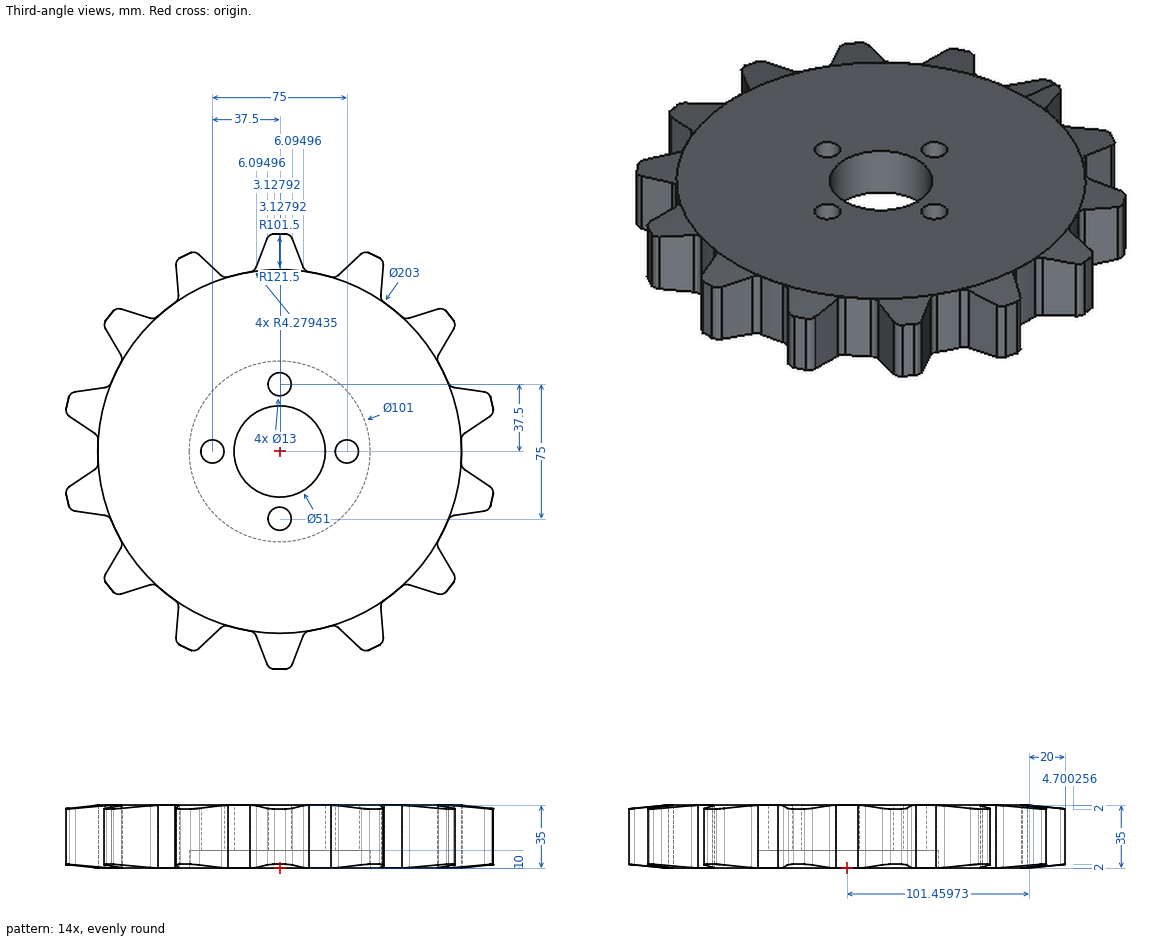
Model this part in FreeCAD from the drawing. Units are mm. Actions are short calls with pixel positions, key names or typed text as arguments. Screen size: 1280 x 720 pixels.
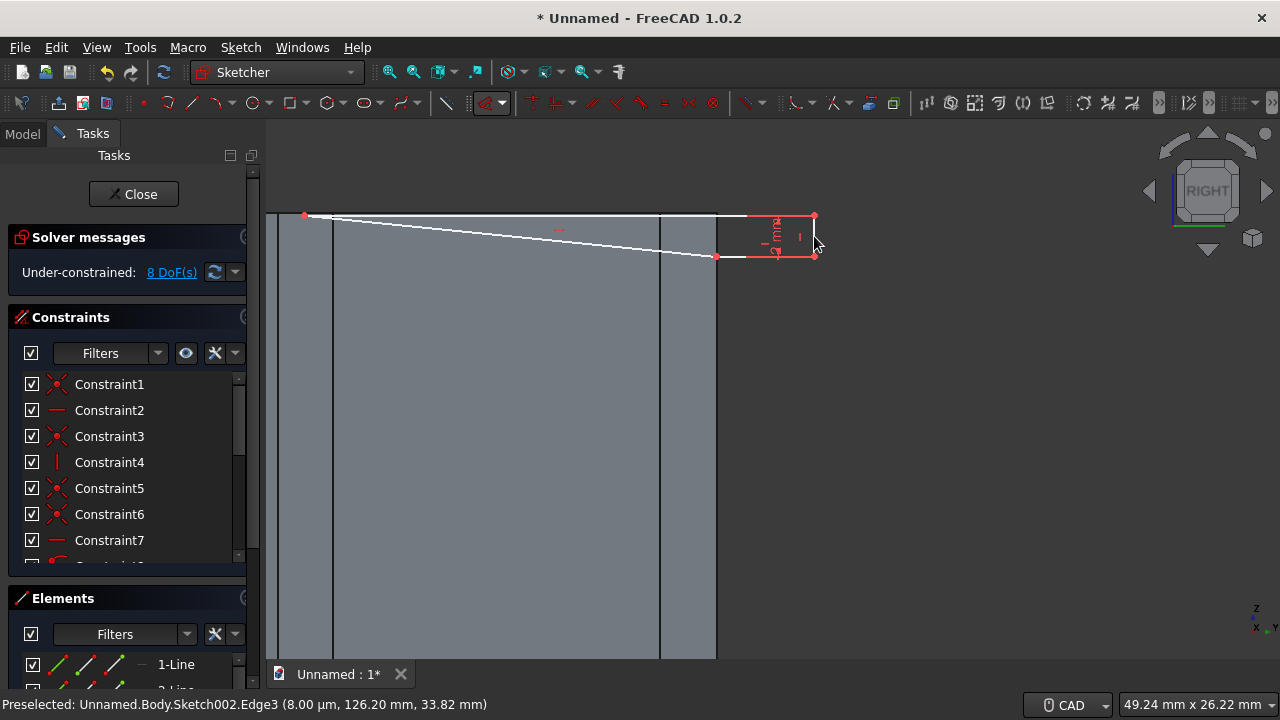
scroll(823, 239, down, 4)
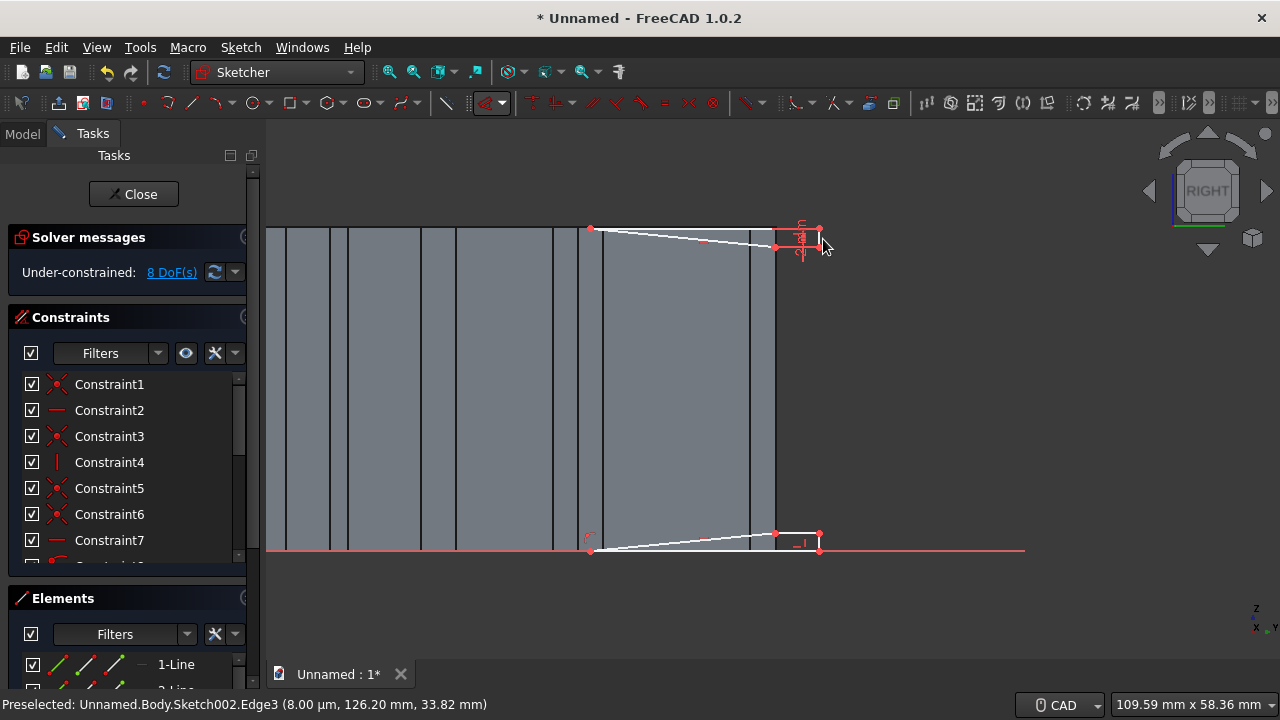
scroll(819, 546, up, 5)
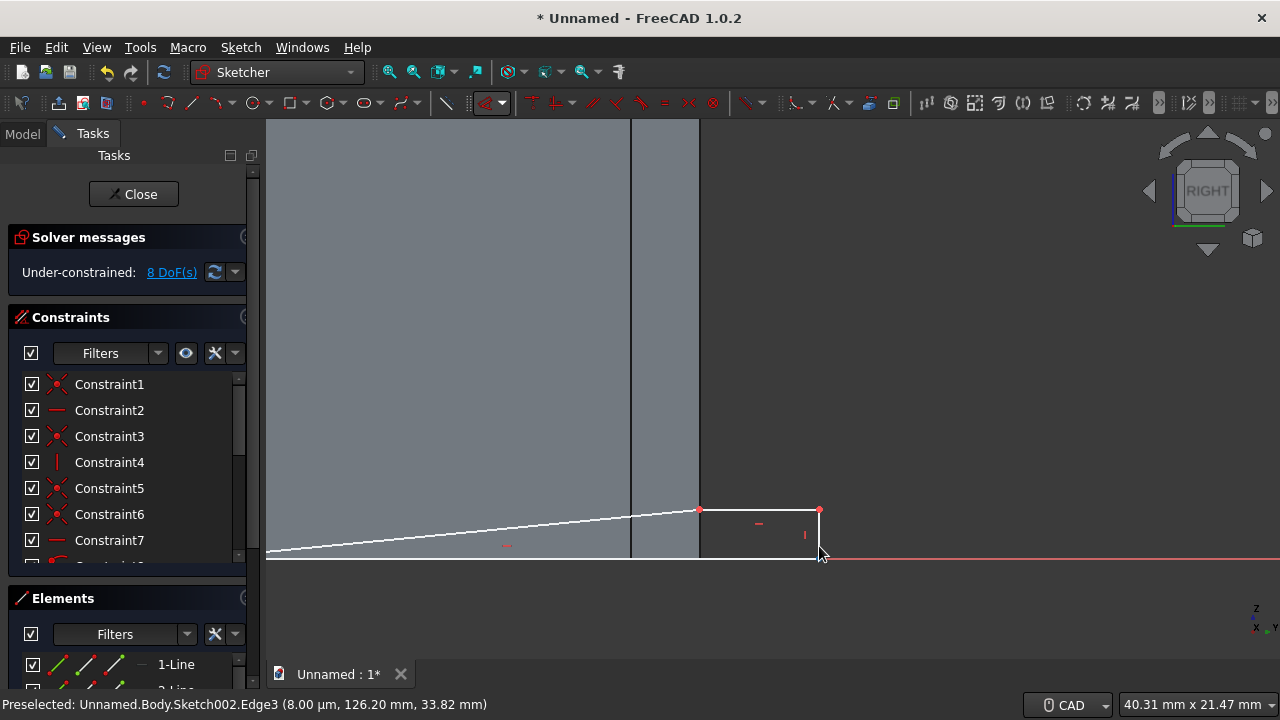
click(819, 544)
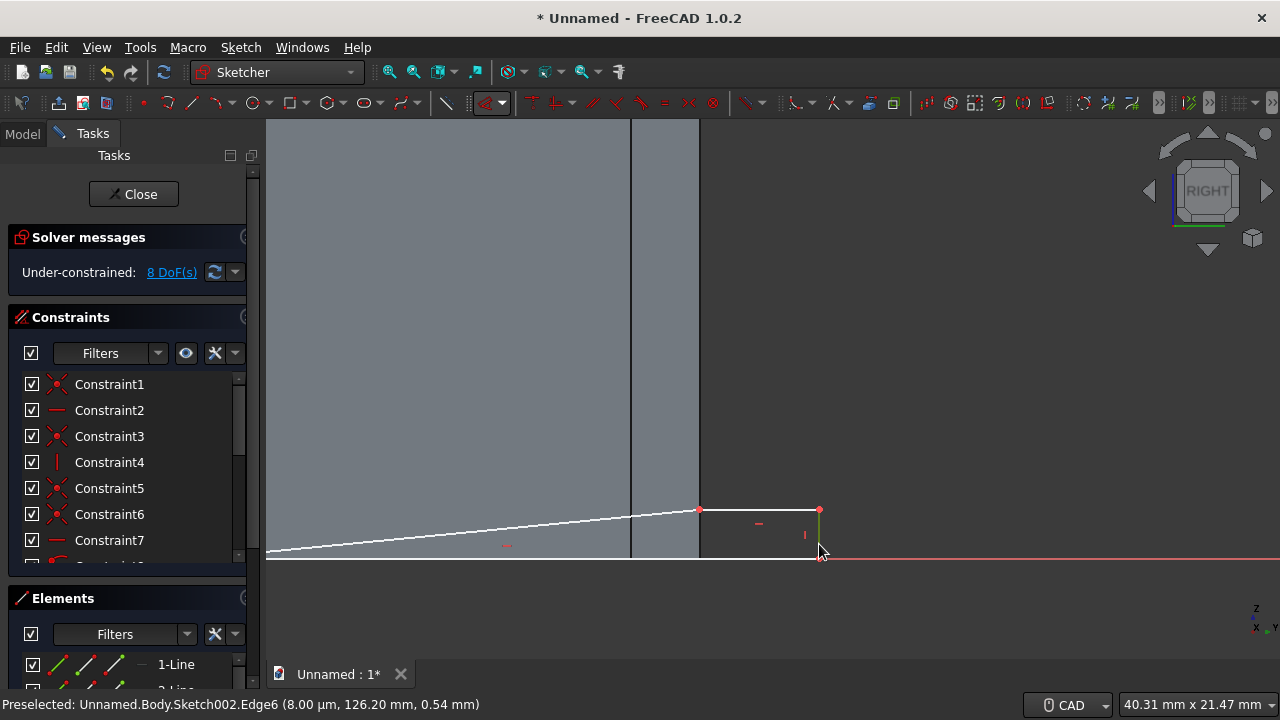
click(504, 104)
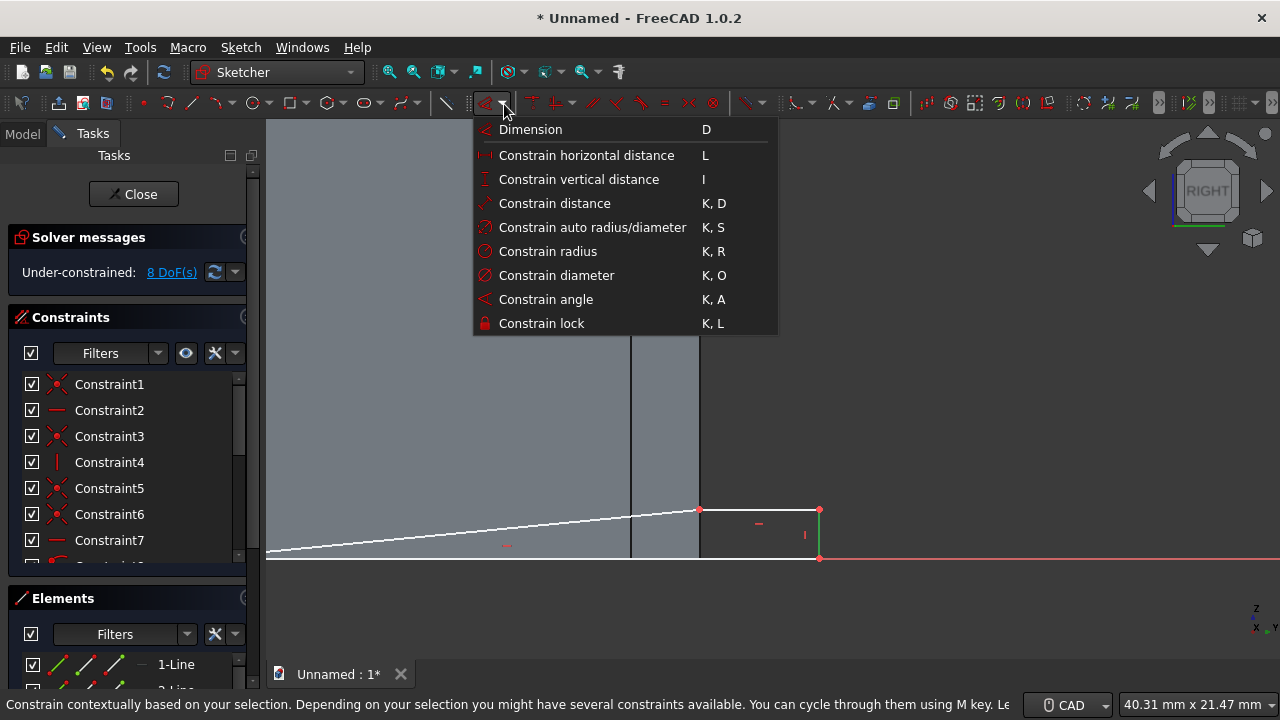
click(626, 179)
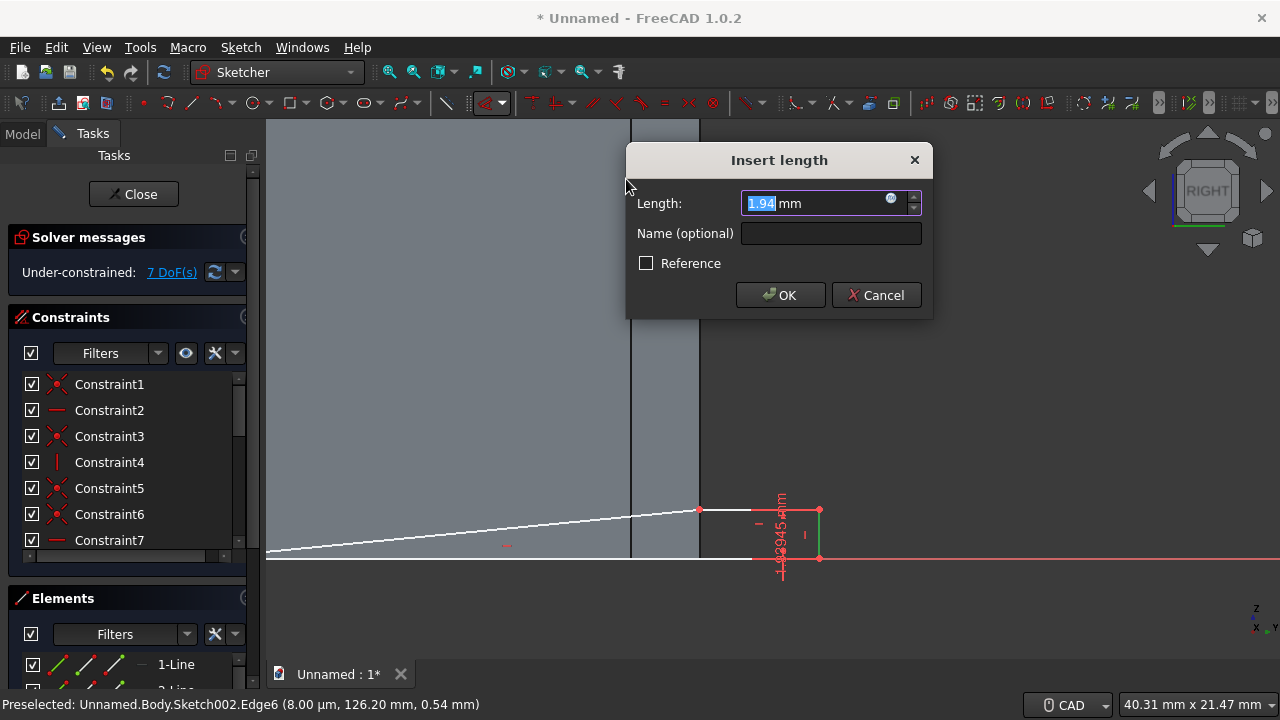
text(2)
key(Return)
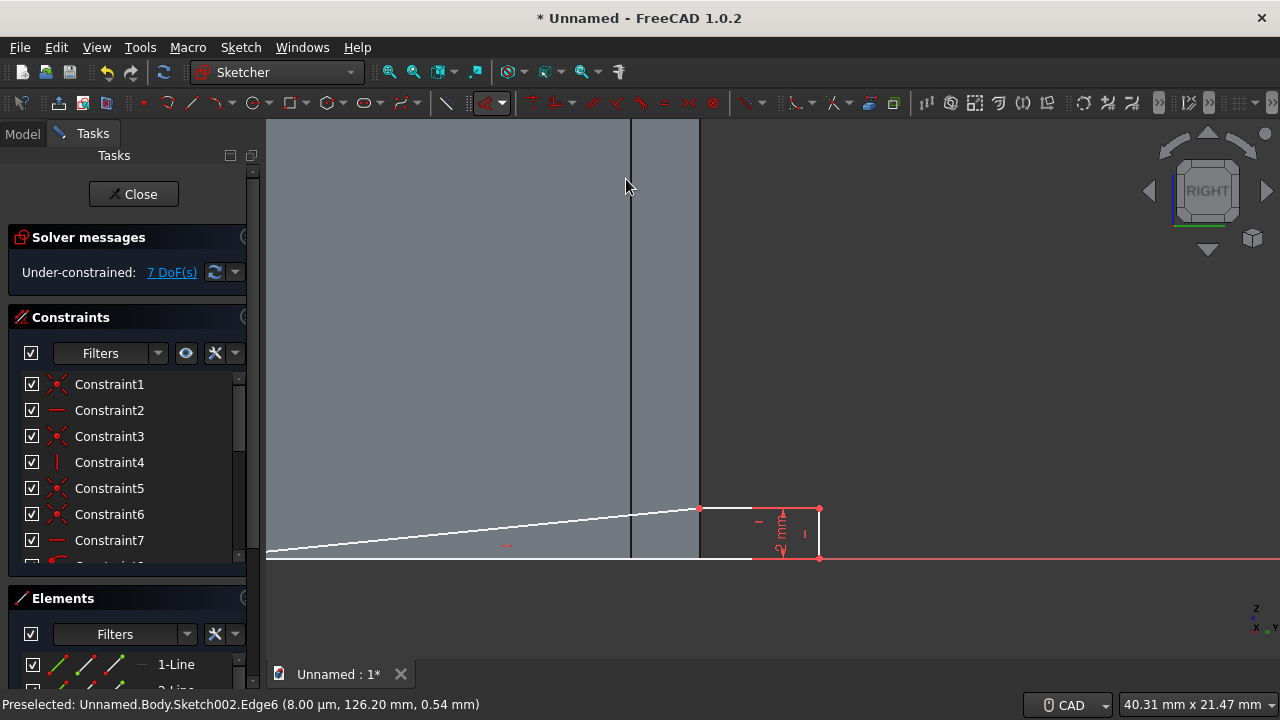
scroll(819, 546, down, 5)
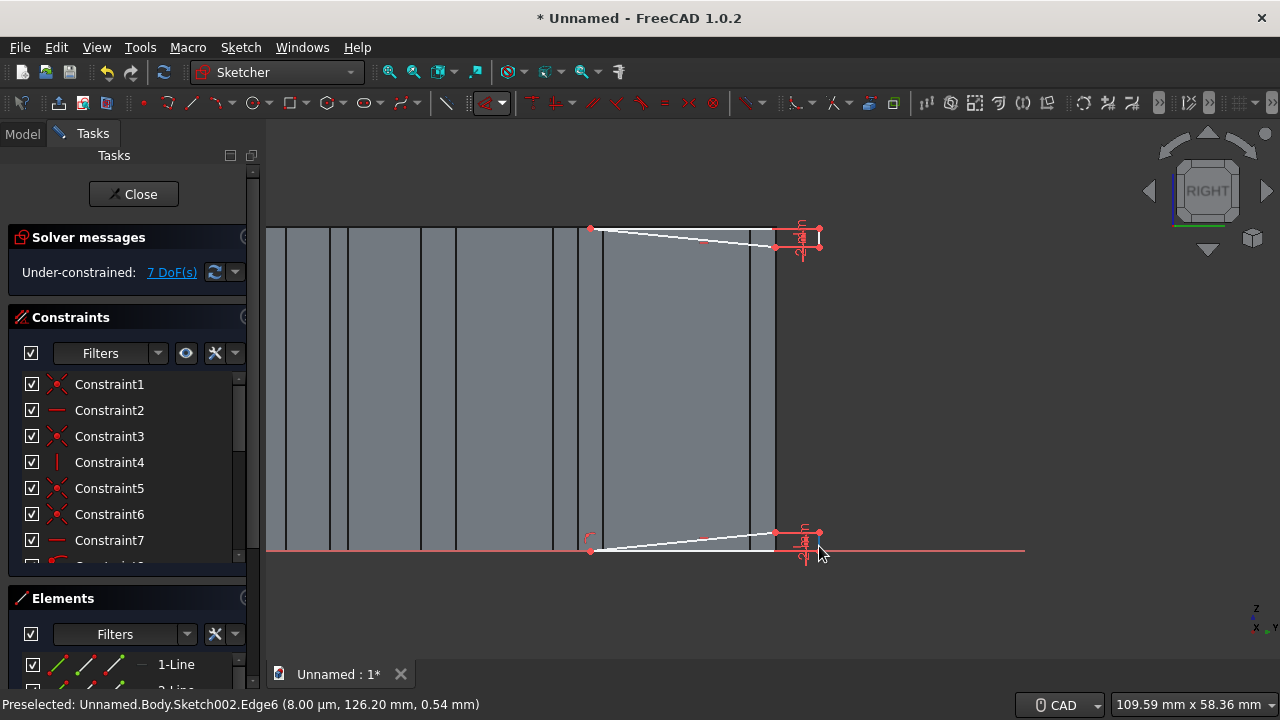
click(590, 229)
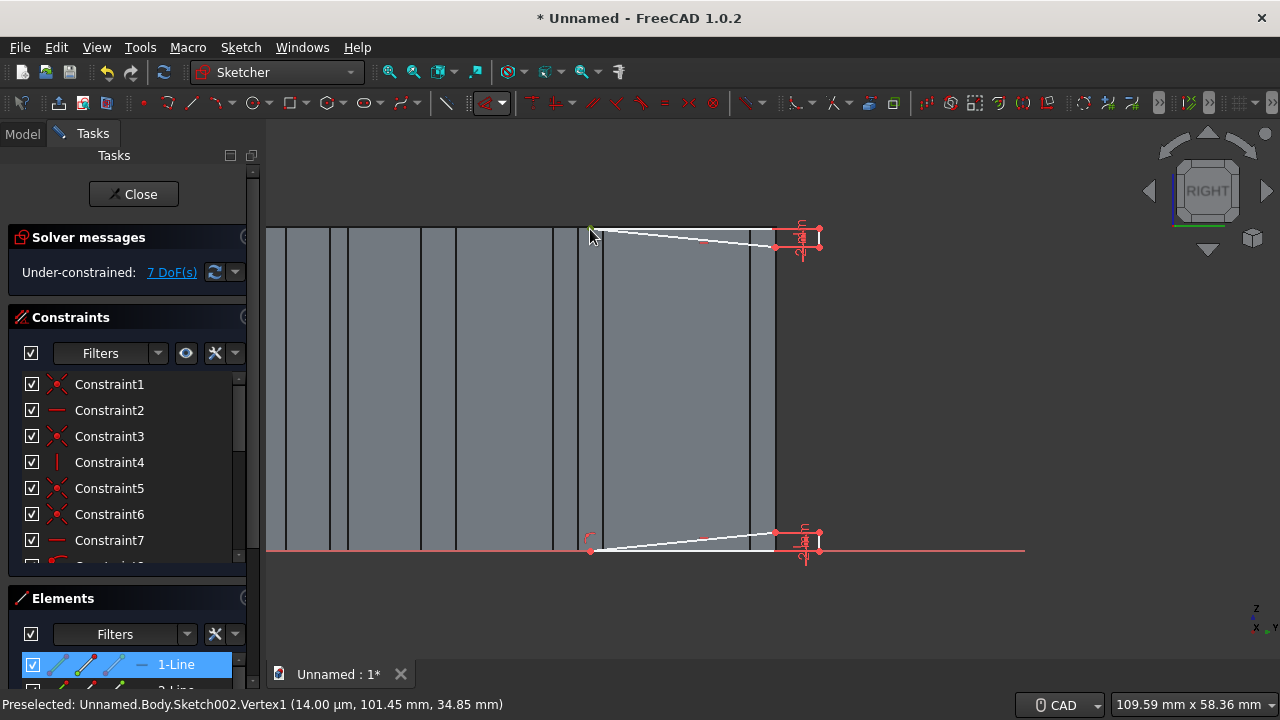
key(i)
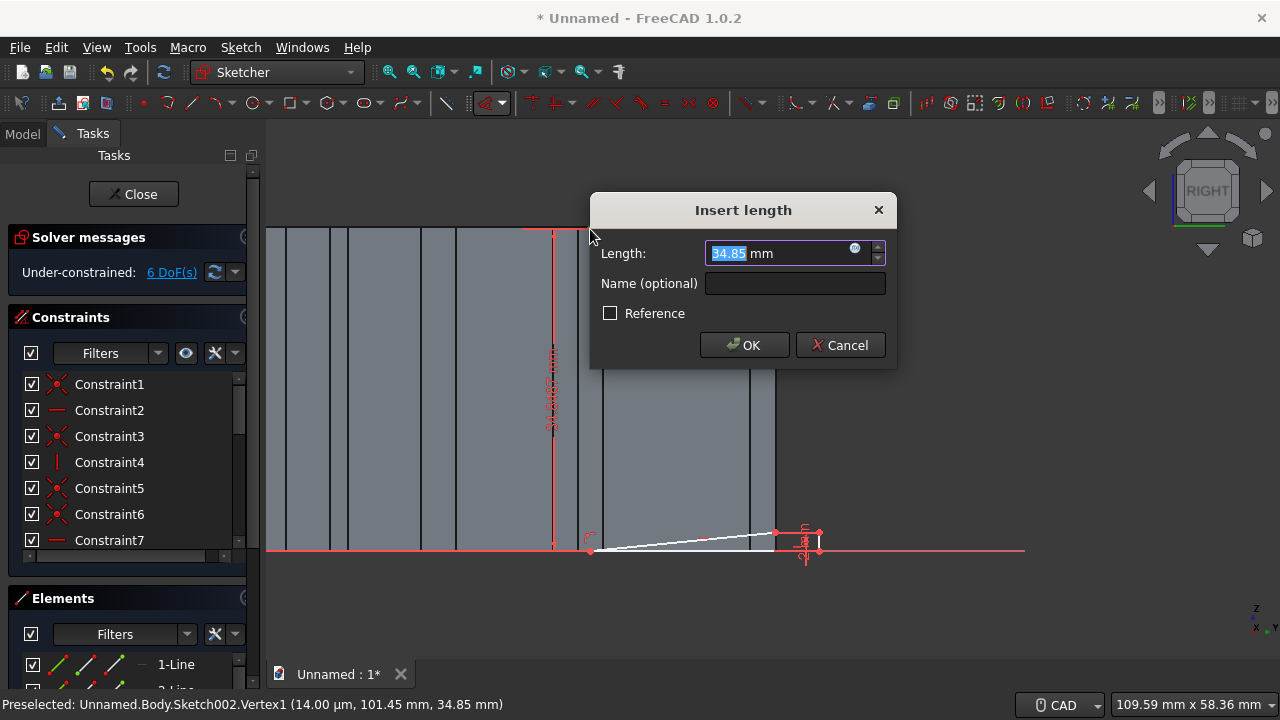
text(35)
key(Return)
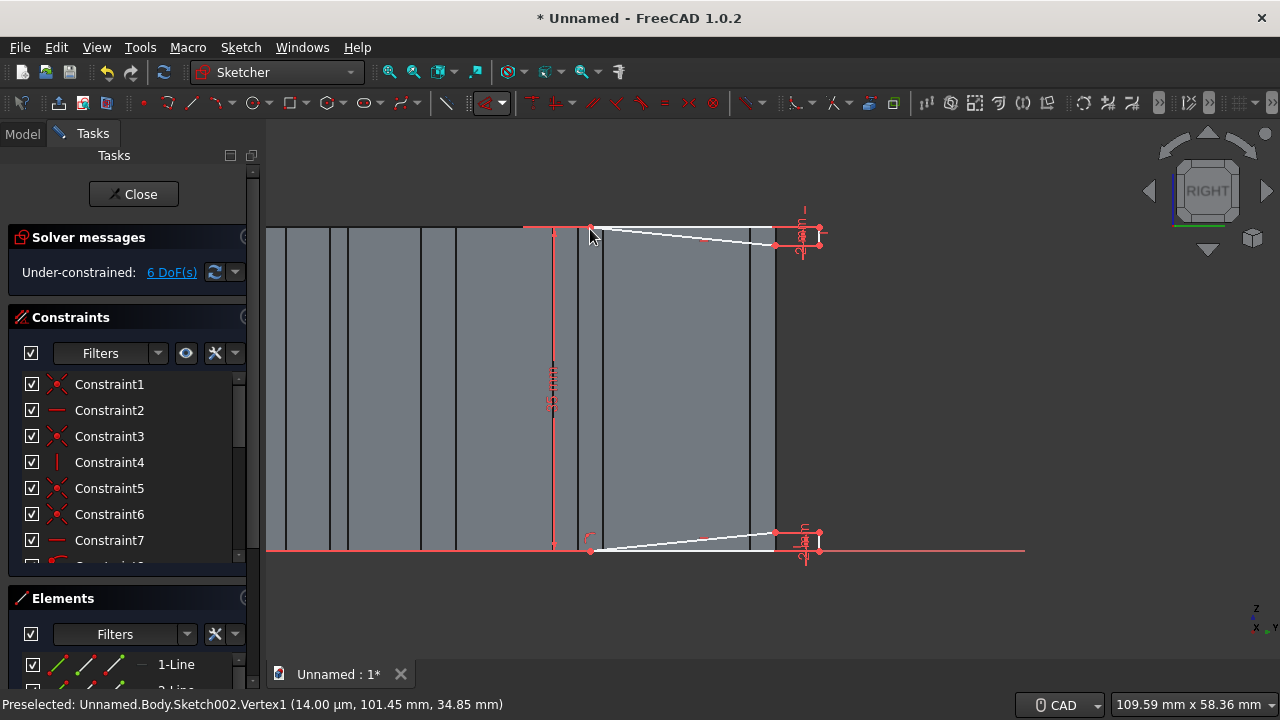
click(720, 240)